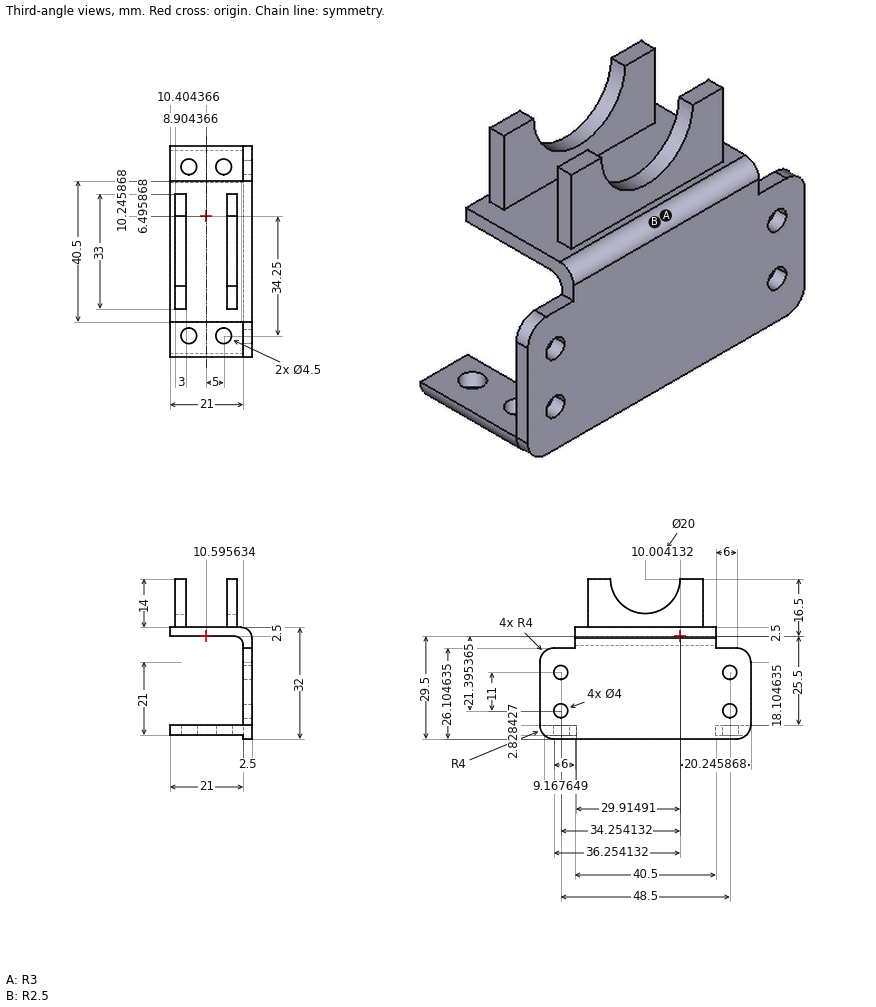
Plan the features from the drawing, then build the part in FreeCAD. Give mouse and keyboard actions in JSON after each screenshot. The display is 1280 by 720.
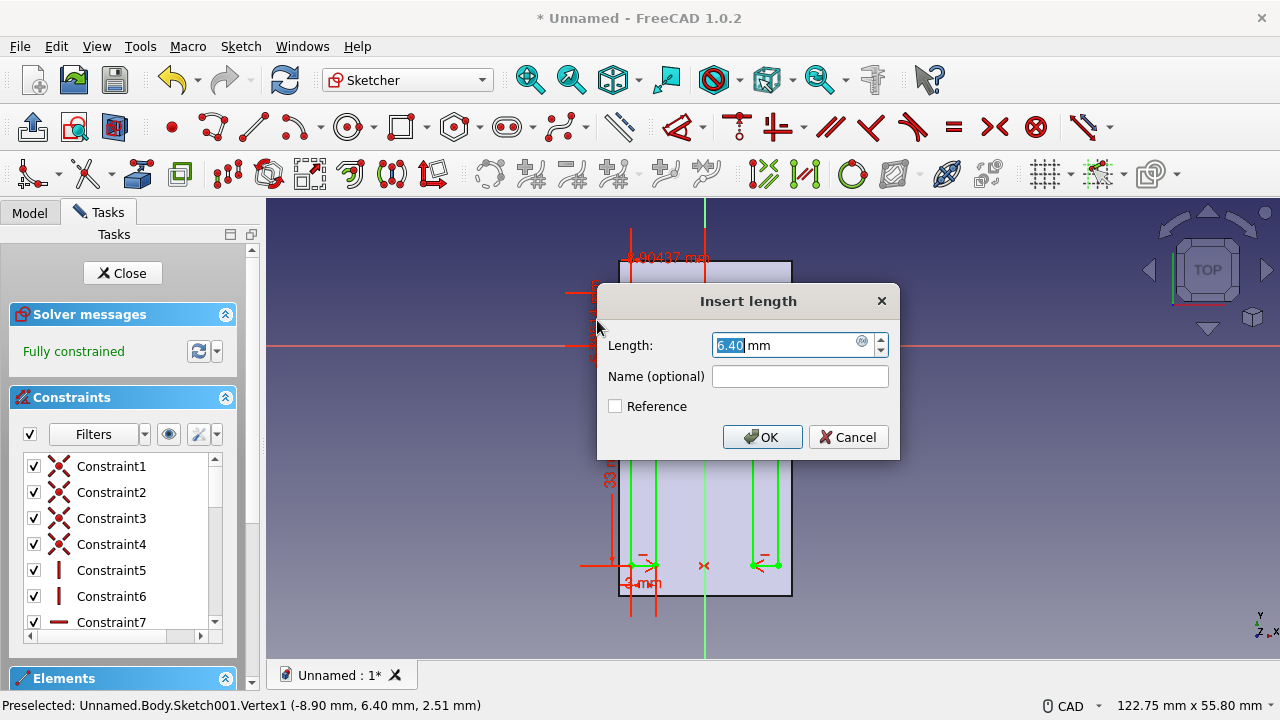
{"action": "type", "text": "6.495868"}
{"action": "key", "text": "Return"}
{"action": "key", "text": "Escape"}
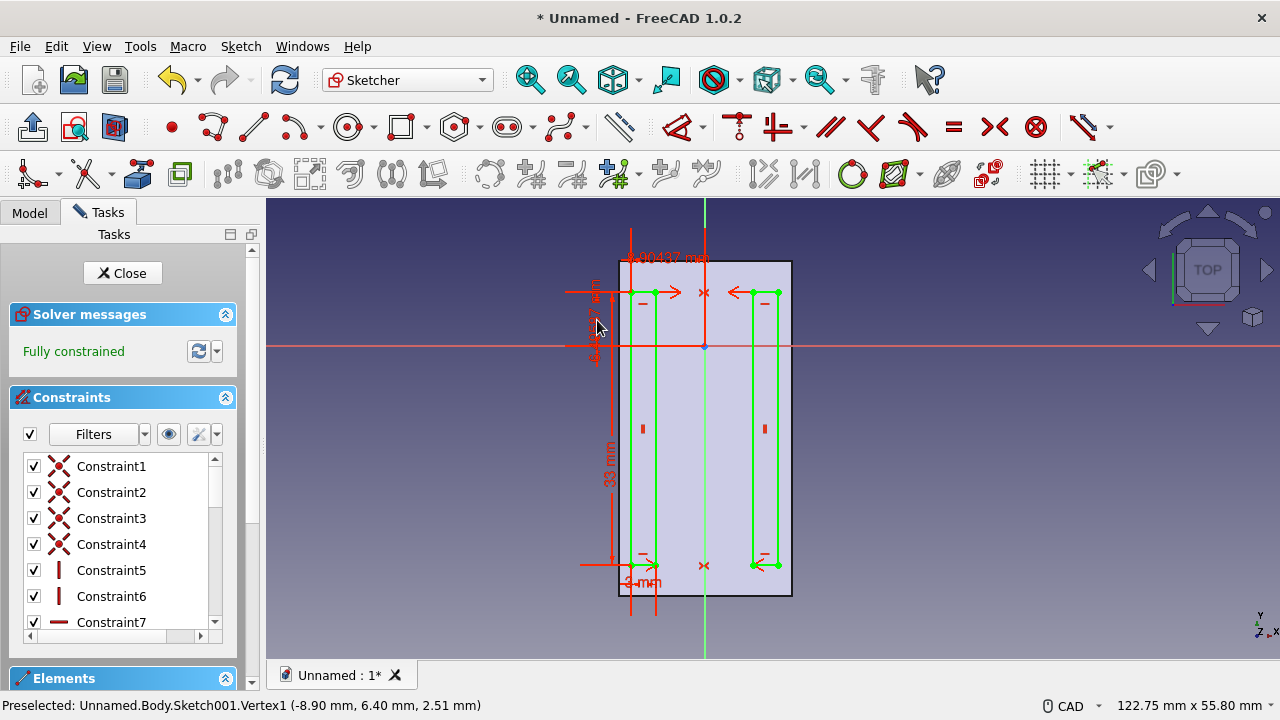
{"action": "left_click", "coordinate": [123, 273]}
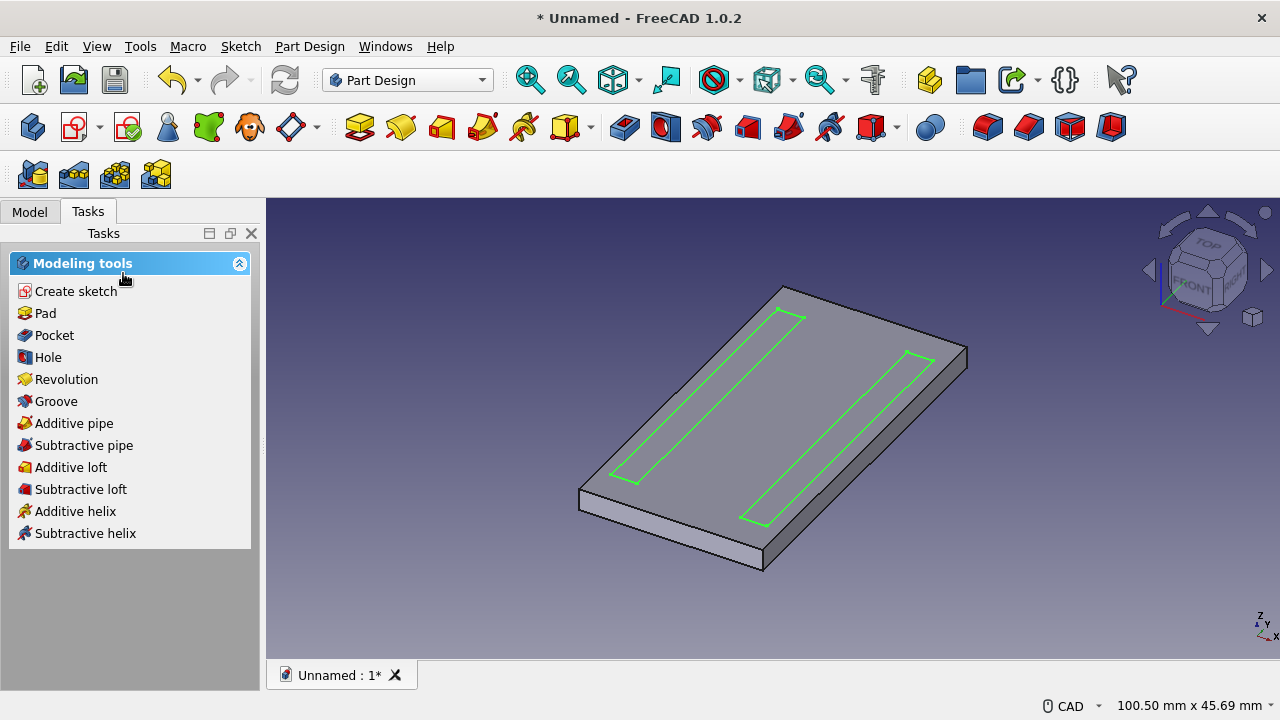
{"action": "left_click", "coordinate": [360, 128]}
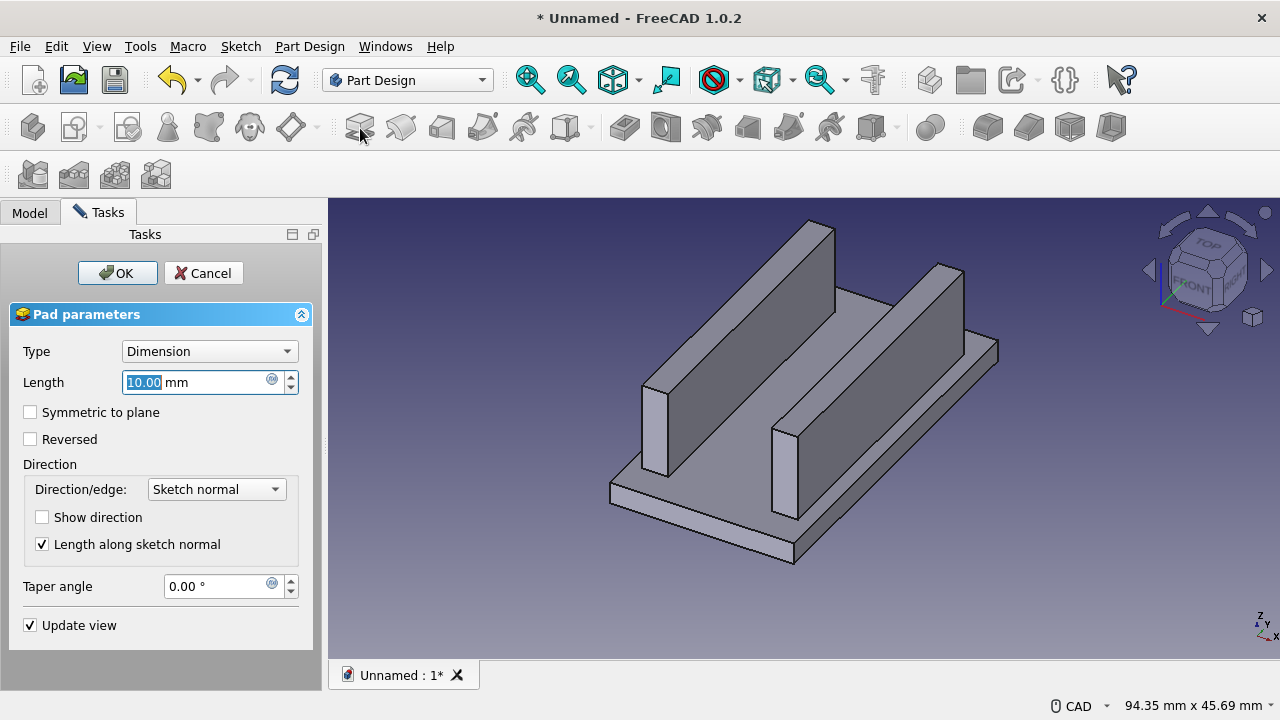
{"action": "type", "text": "14"}
{"action": "key", "text": "Tab"}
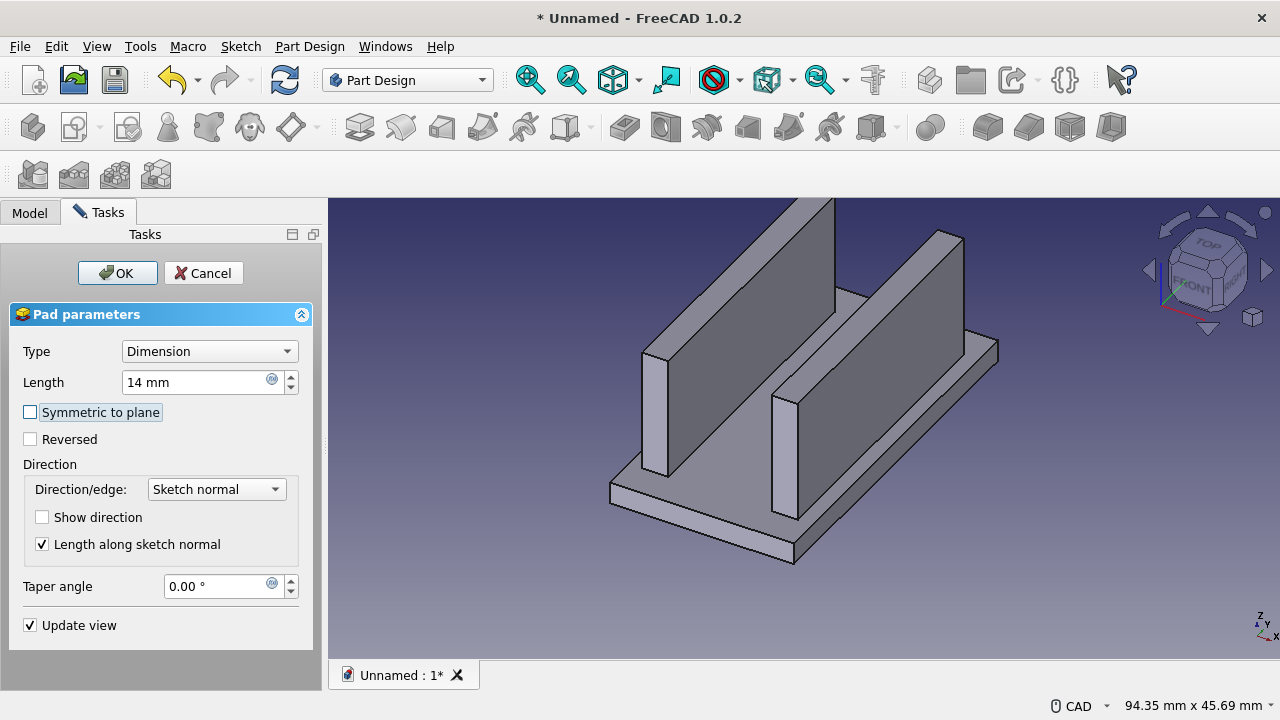
{"action": "left_click", "coordinate": [118, 273]}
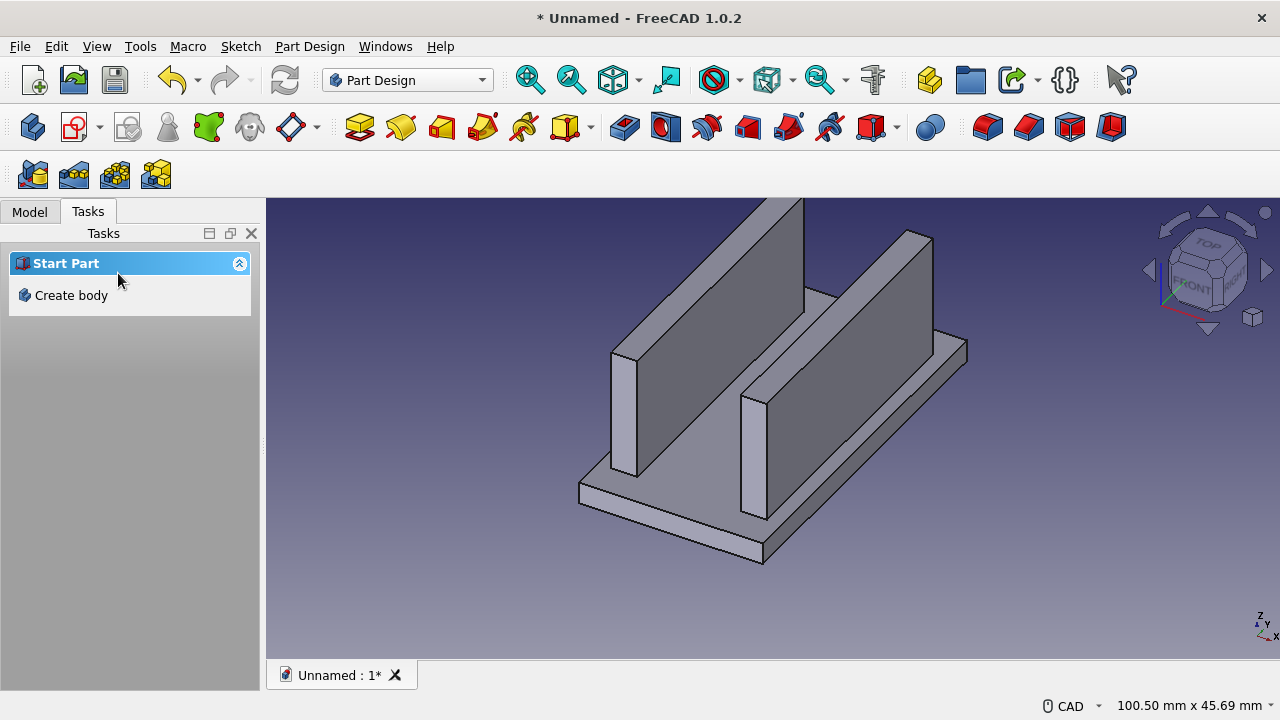
{"action": "left_click", "coordinate": [531, 80]}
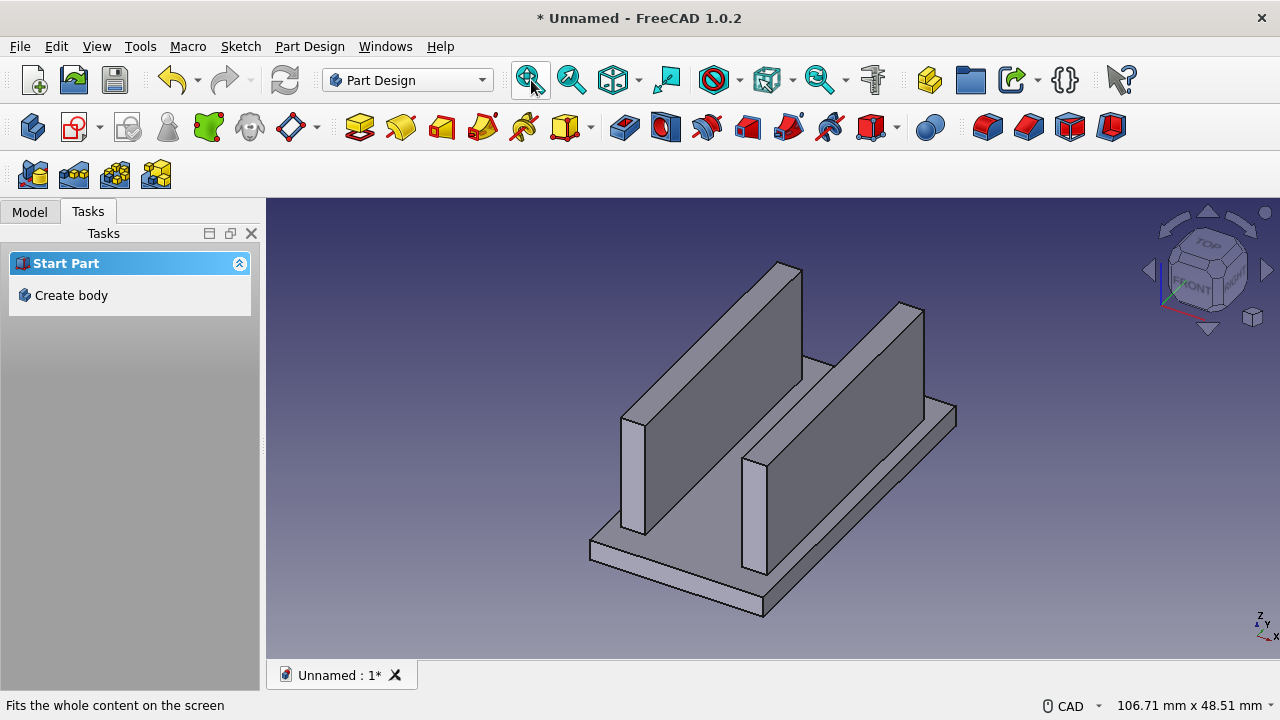
{"action": "left_click", "coordinate": [890, 397]}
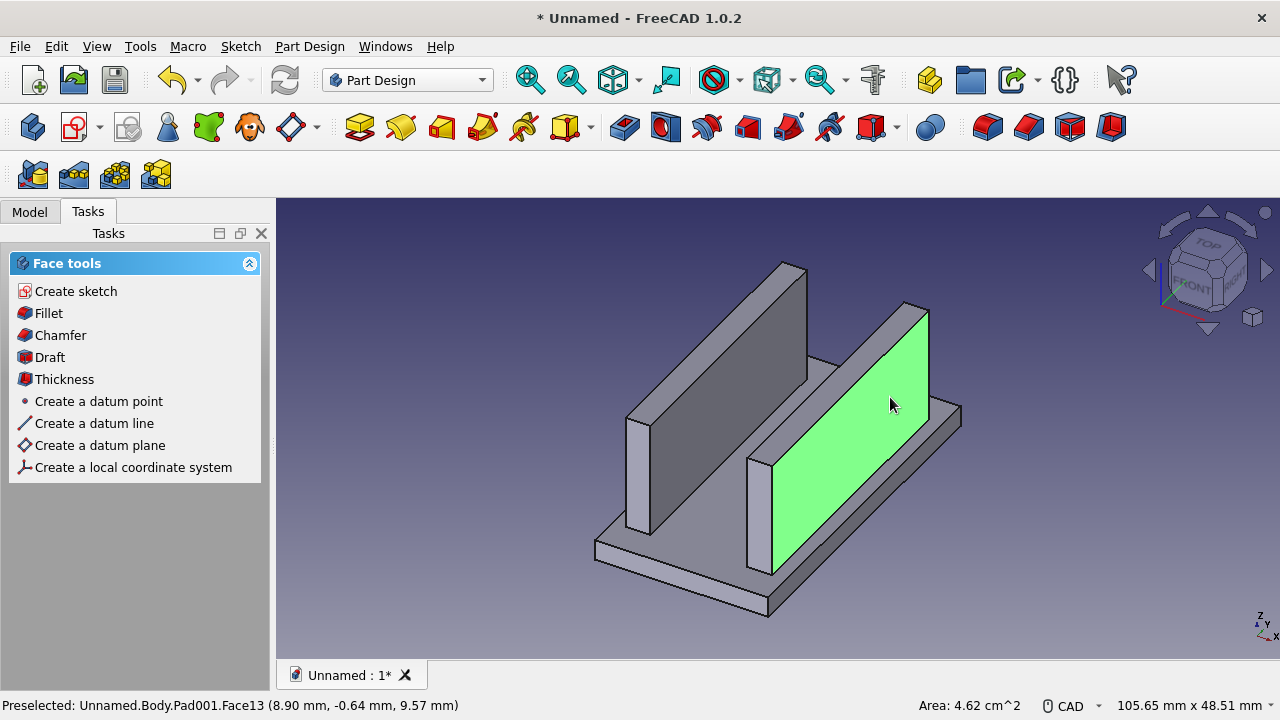
{"action": "left_click", "coordinate": [74, 128]}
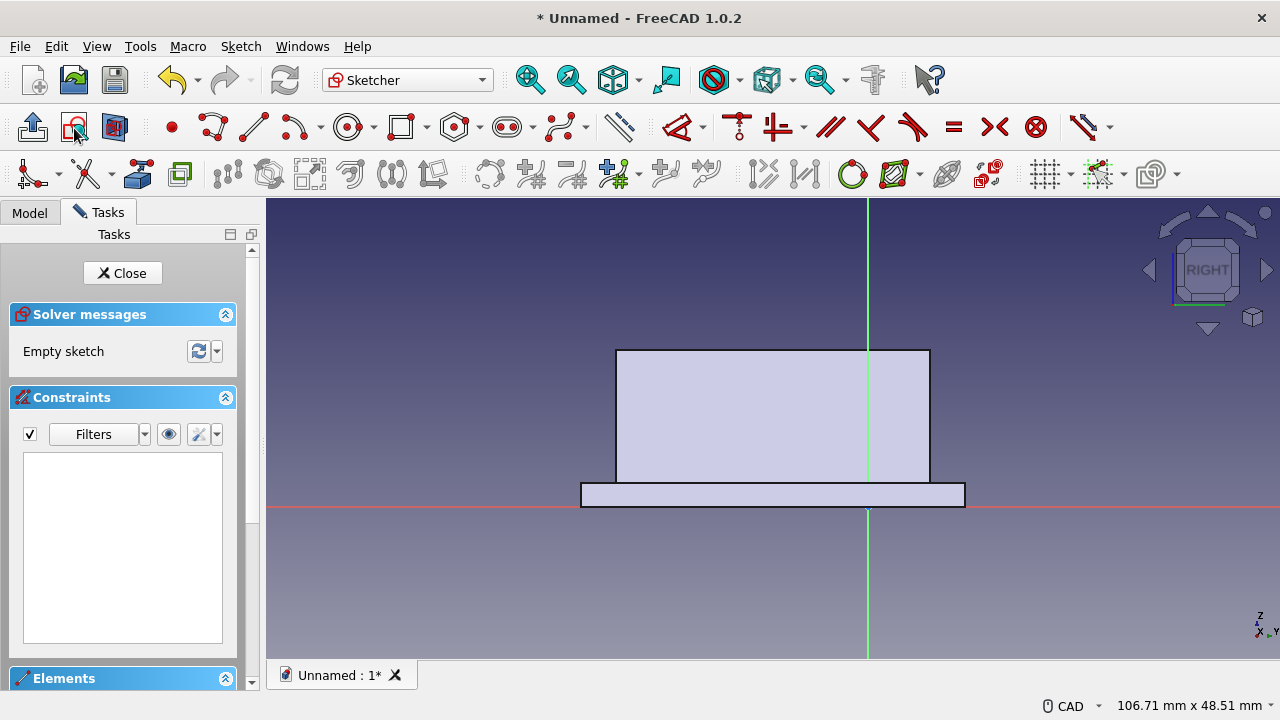
{"action": "key", "text": "g c"}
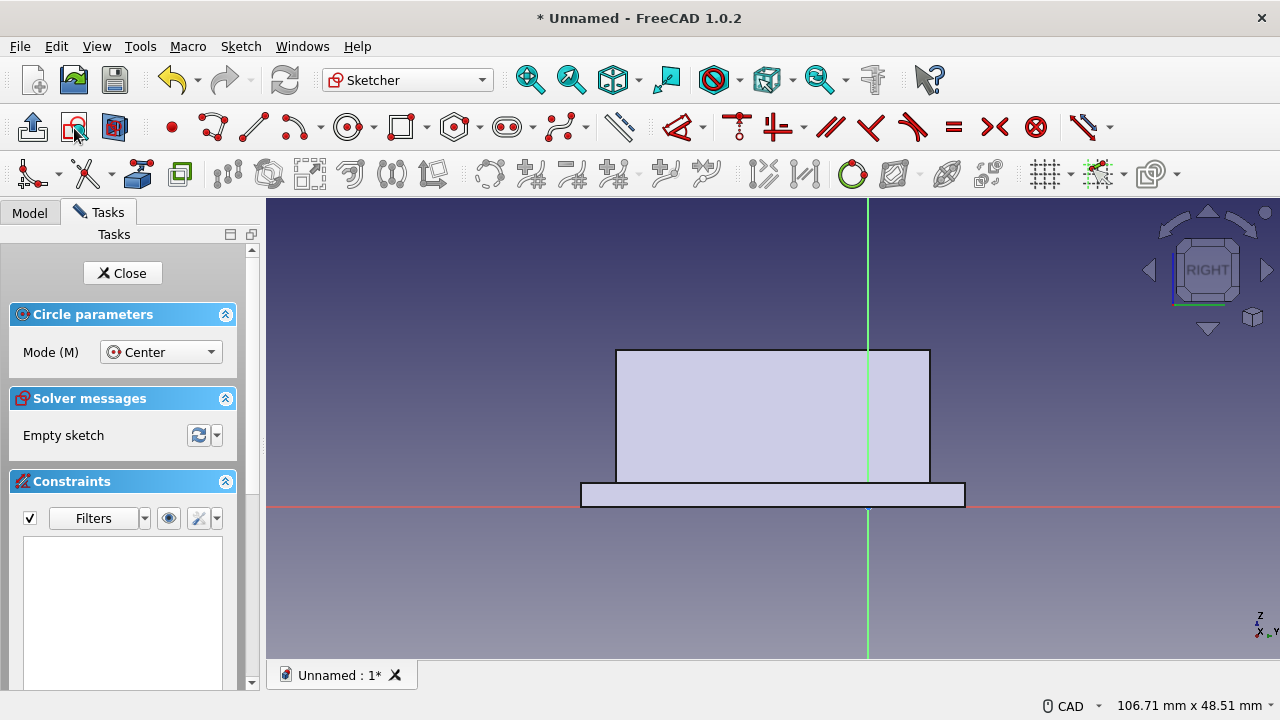
{"action": "left_click", "coordinate": [773, 350]}
{"action": "left_click", "coordinate": [840, 283]}
{"action": "key", "text": "Escape"}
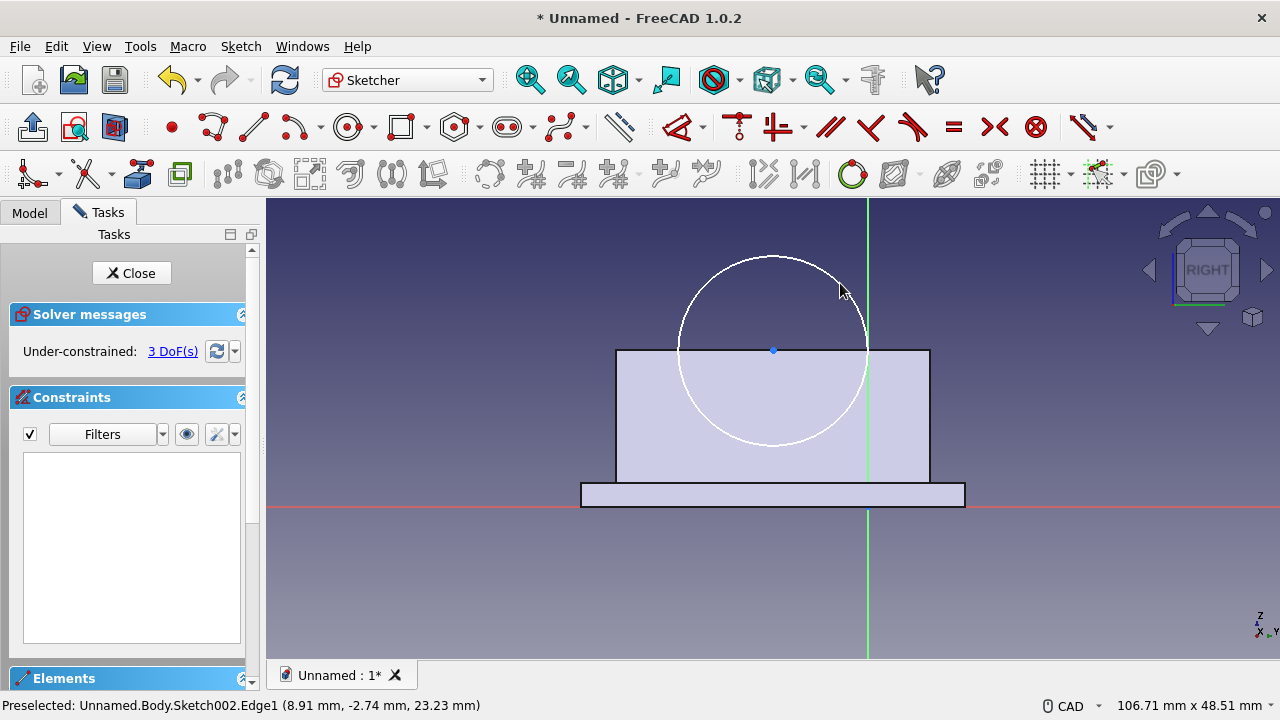
{"action": "left_click", "coordinate": [676, 128]}